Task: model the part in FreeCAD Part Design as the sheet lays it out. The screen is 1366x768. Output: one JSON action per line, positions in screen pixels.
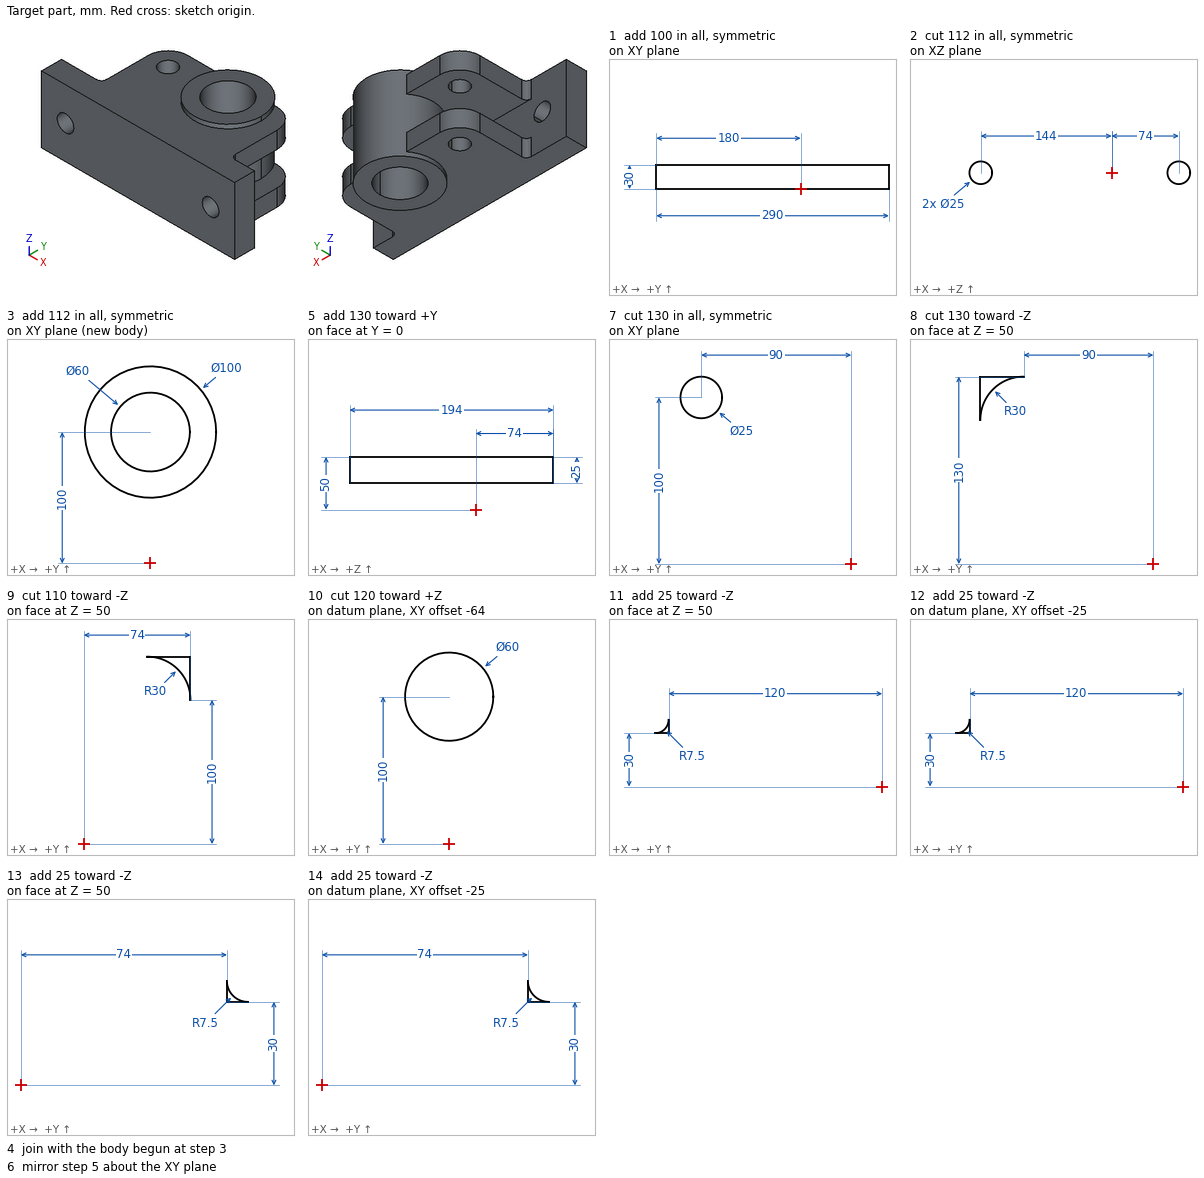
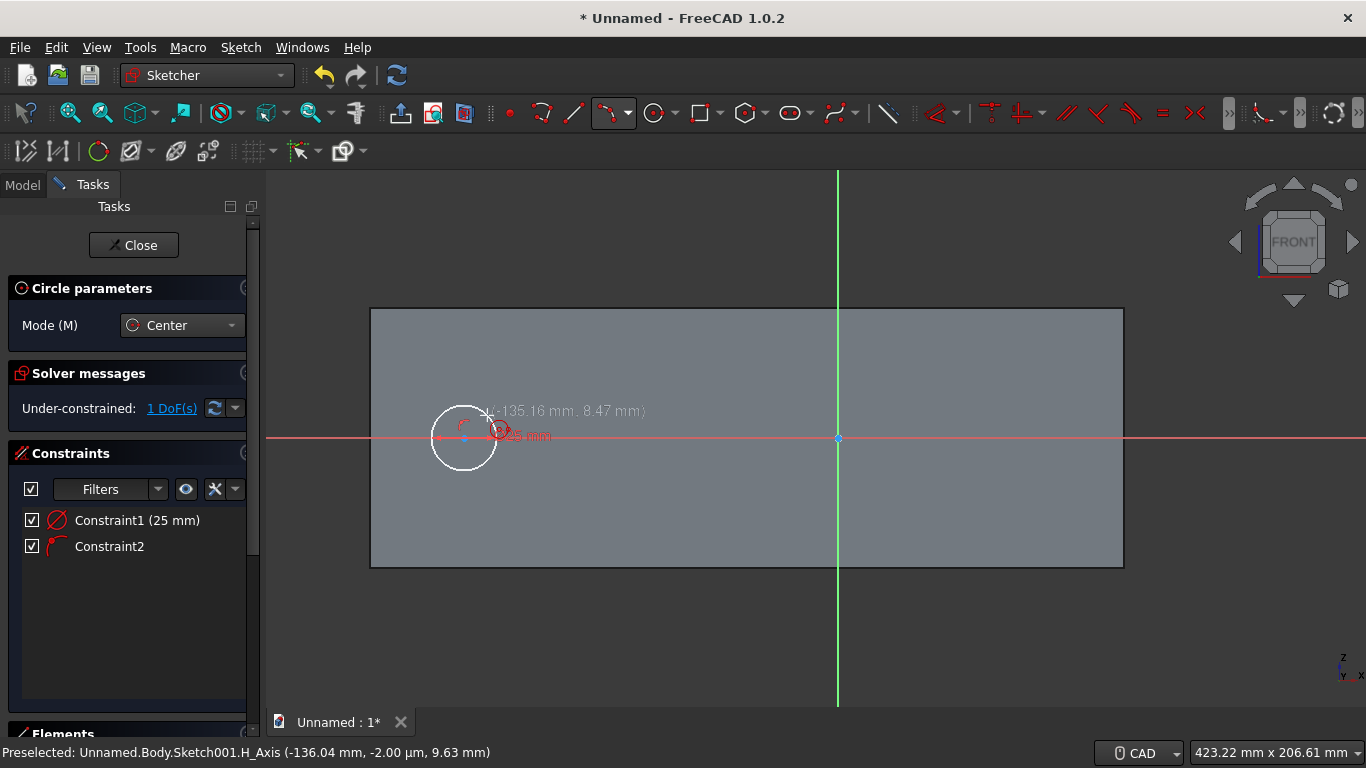
{"action": "left_click", "coordinate": [1031, 438]}
{"action": "mouse_move", "coordinate": [1054, 415]}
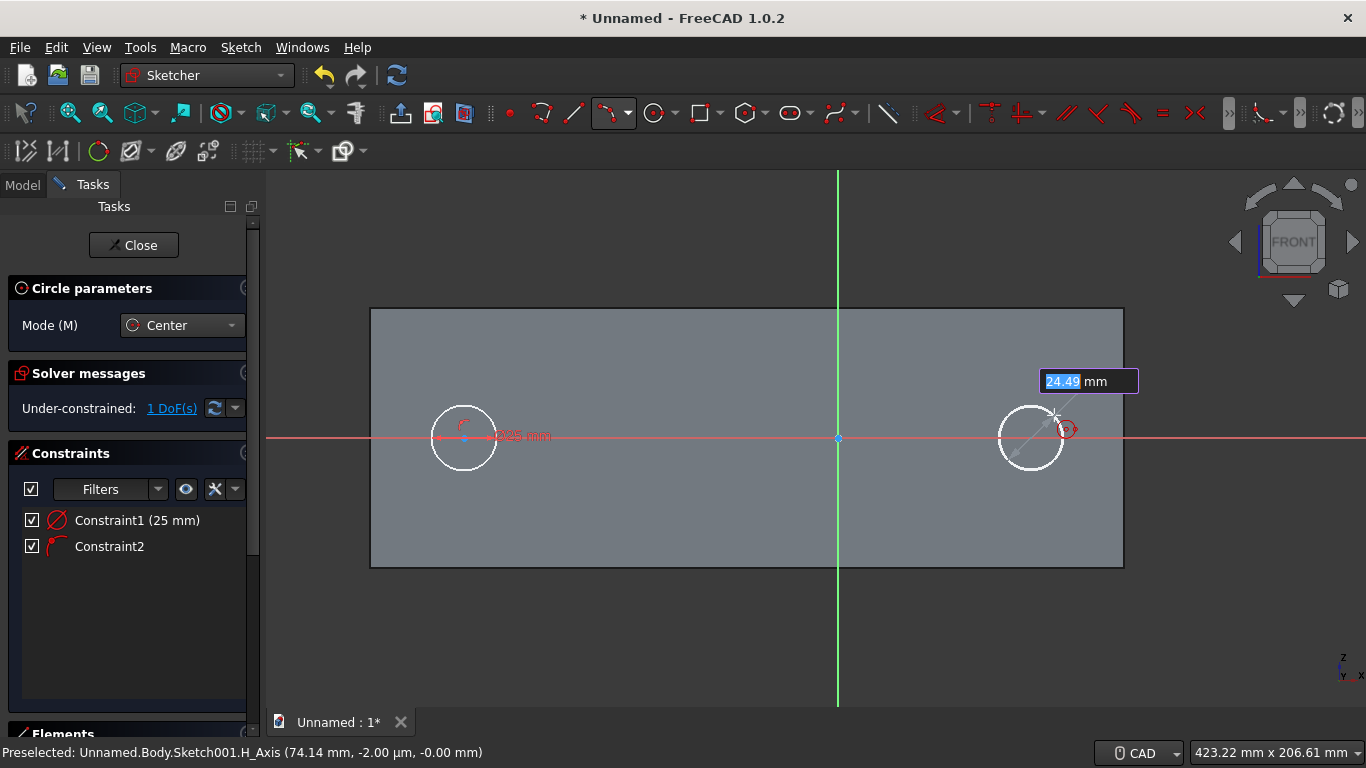
{"action": "type", "text": "25"}
{"action": "key", "text": "Return"}
{"action": "key", "text": "Escape"}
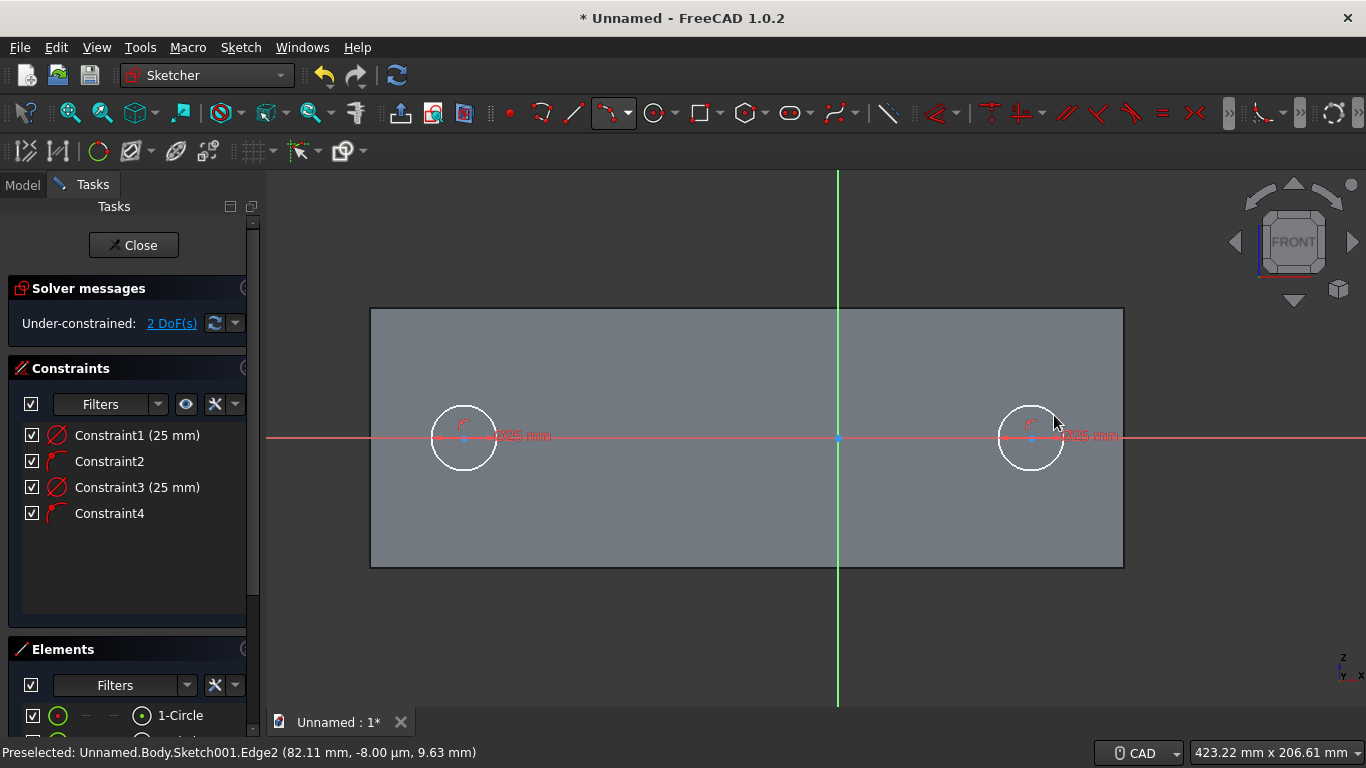
{"action": "left_click", "coordinate": [936, 114]}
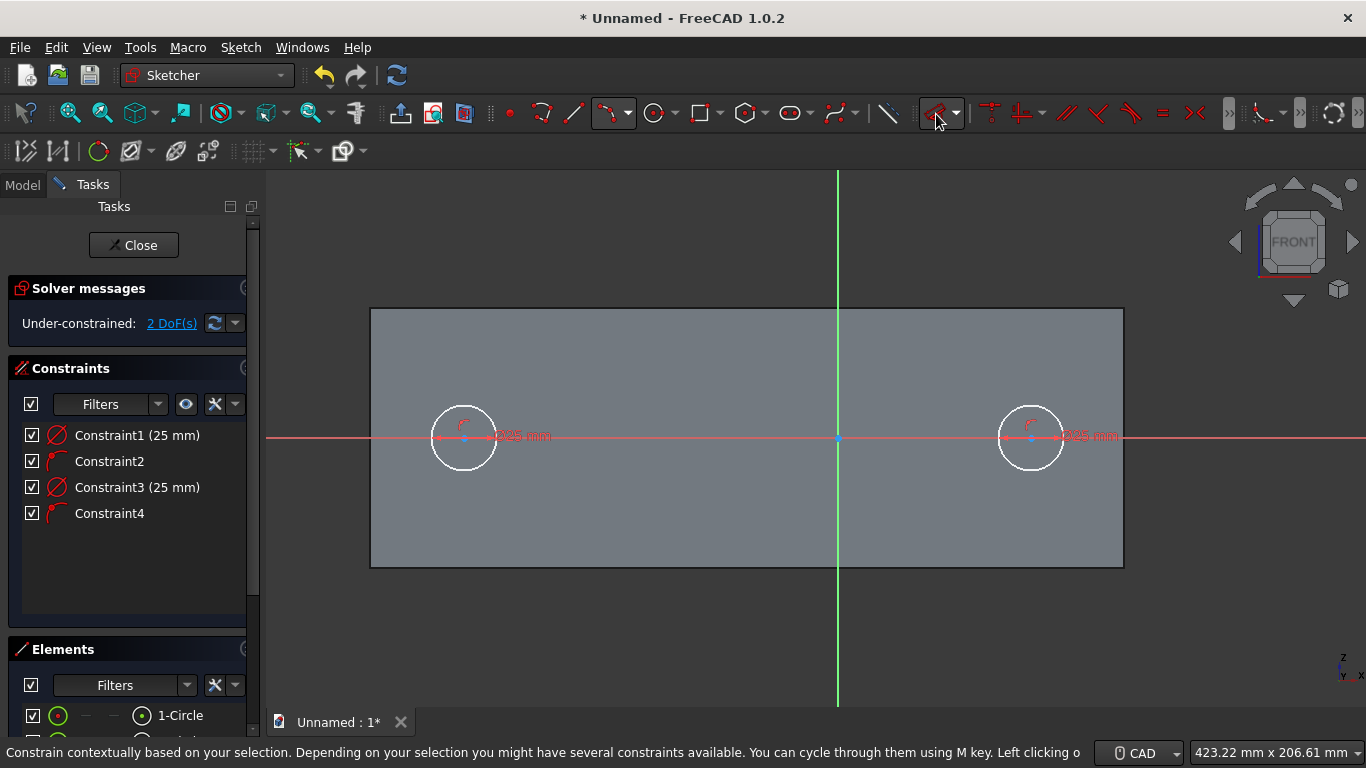
{"action": "left_click", "coordinate": [1031, 438]}
{"action": "left_click", "coordinate": [935, 472]}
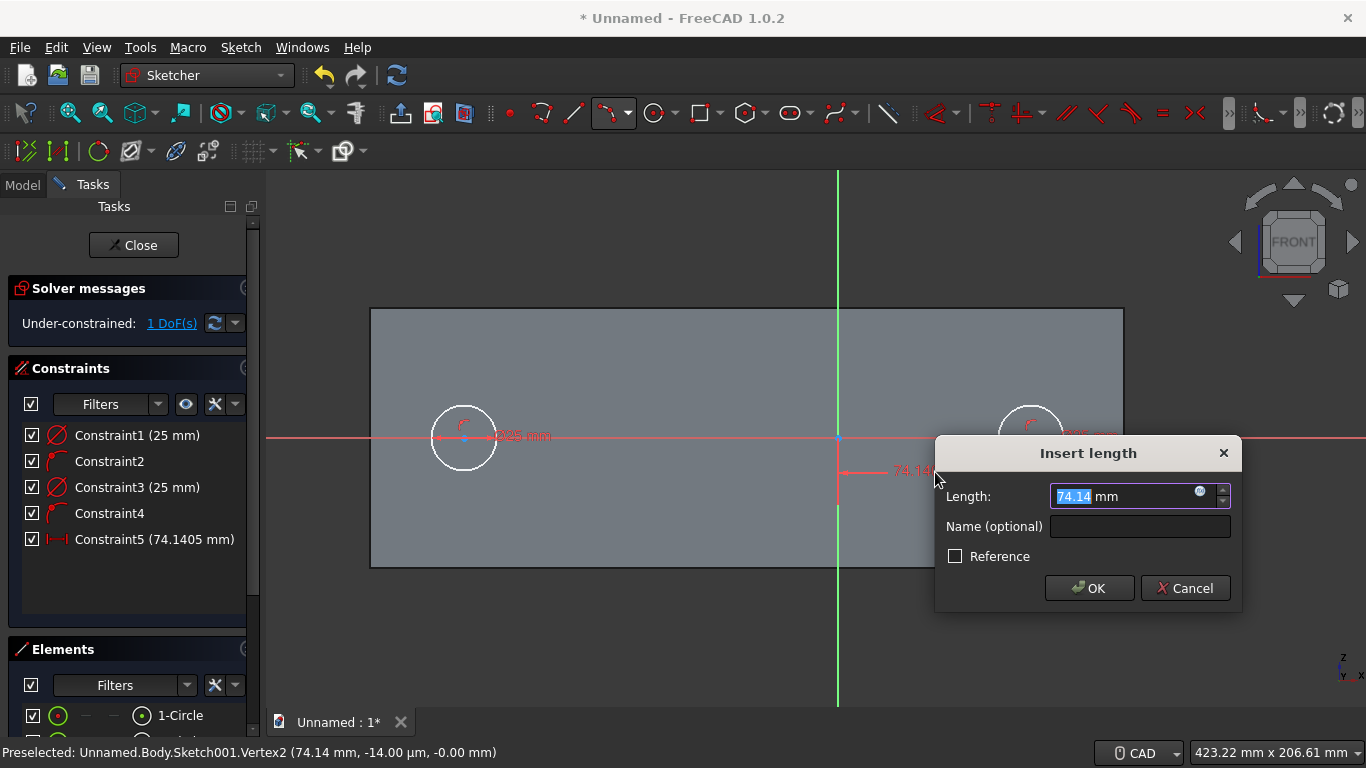
{"action": "type", "text": "74"}
{"action": "key", "text": "Return"}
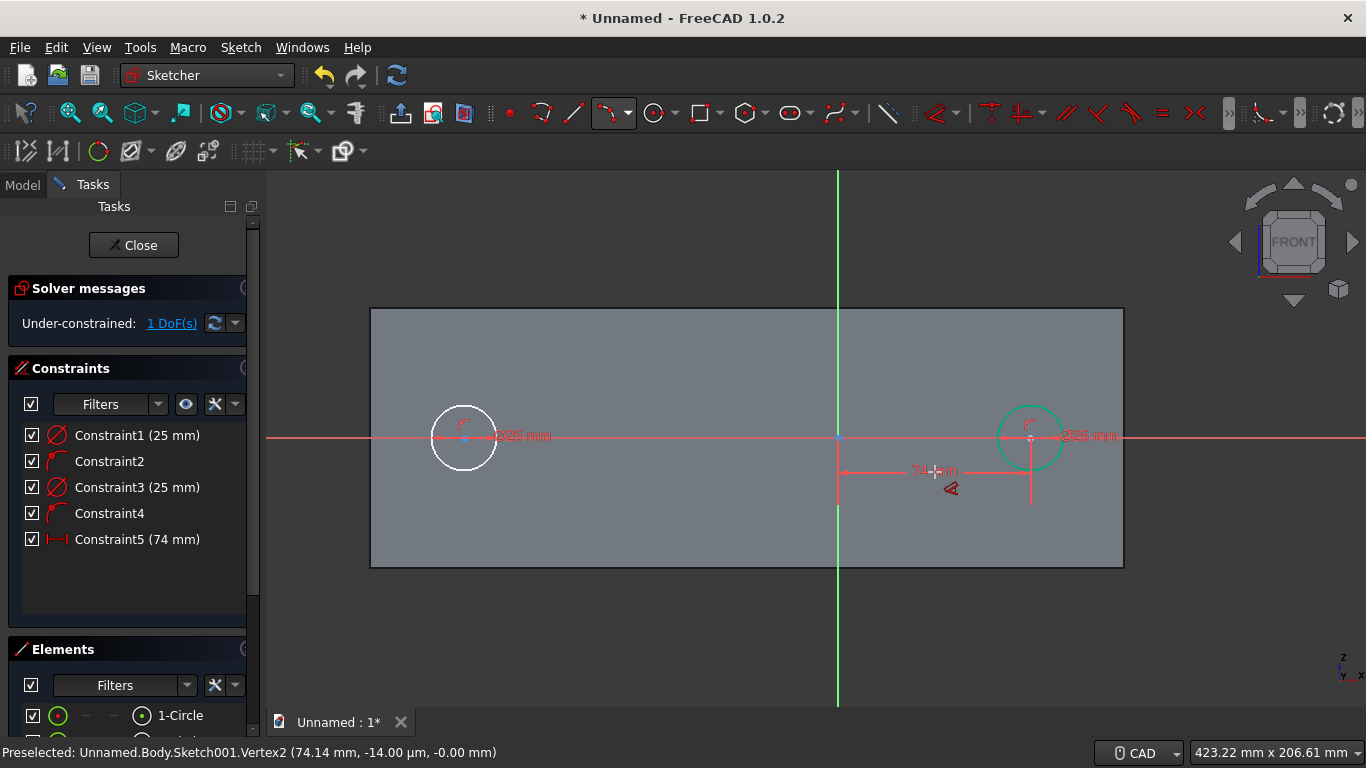
{"action": "left_click", "coordinate": [464, 438]}
{"action": "left_click", "coordinate": [651, 472]}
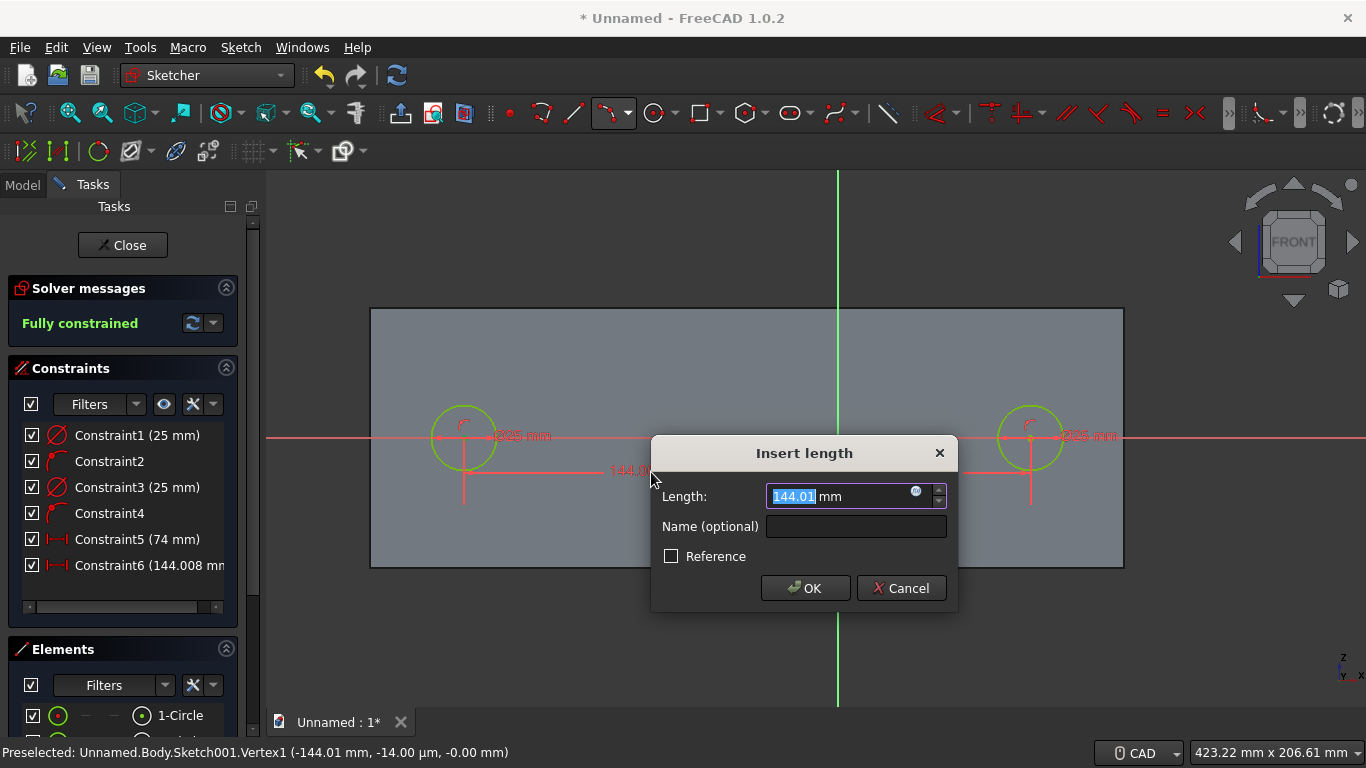
{"action": "type", "text": "144"}
{"action": "key", "text": "Return"}
{"action": "key", "text": "Escape"}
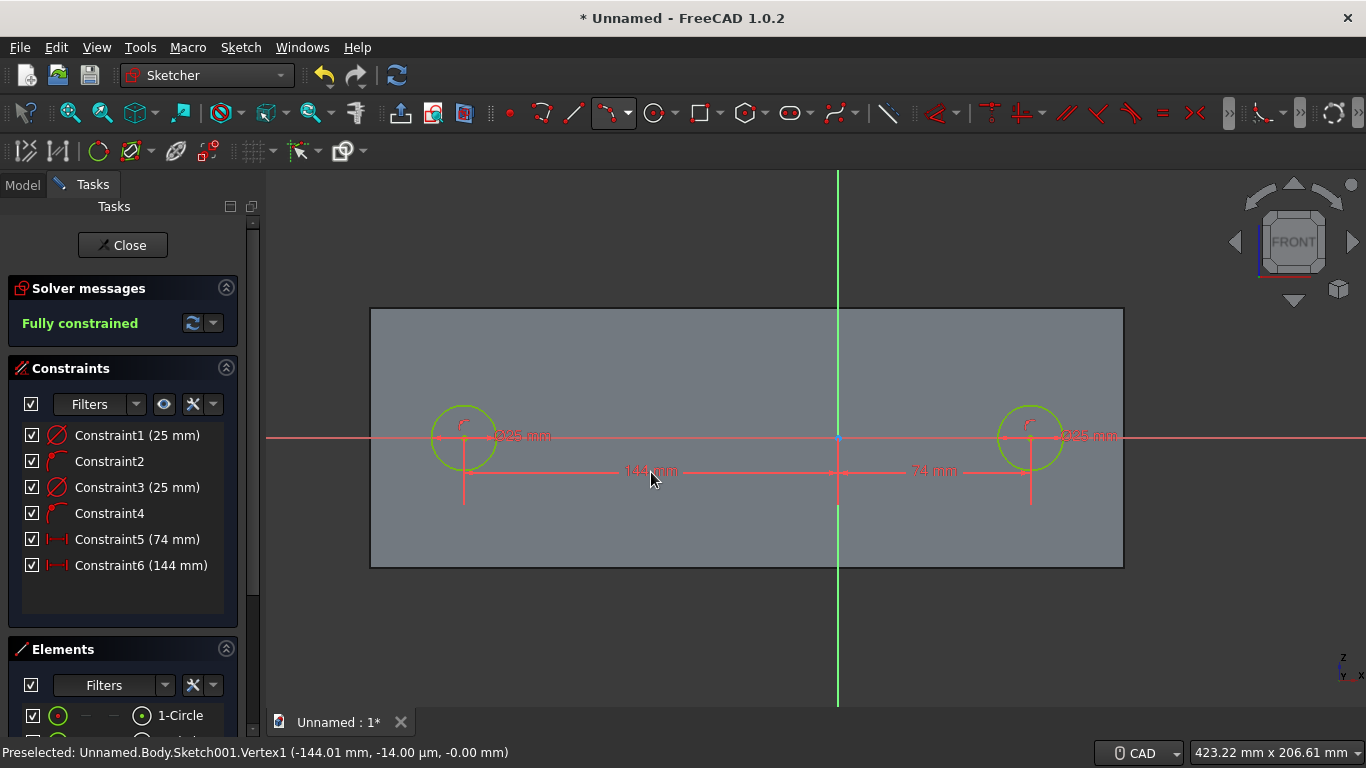
{"action": "left_click", "coordinate": [123, 245]}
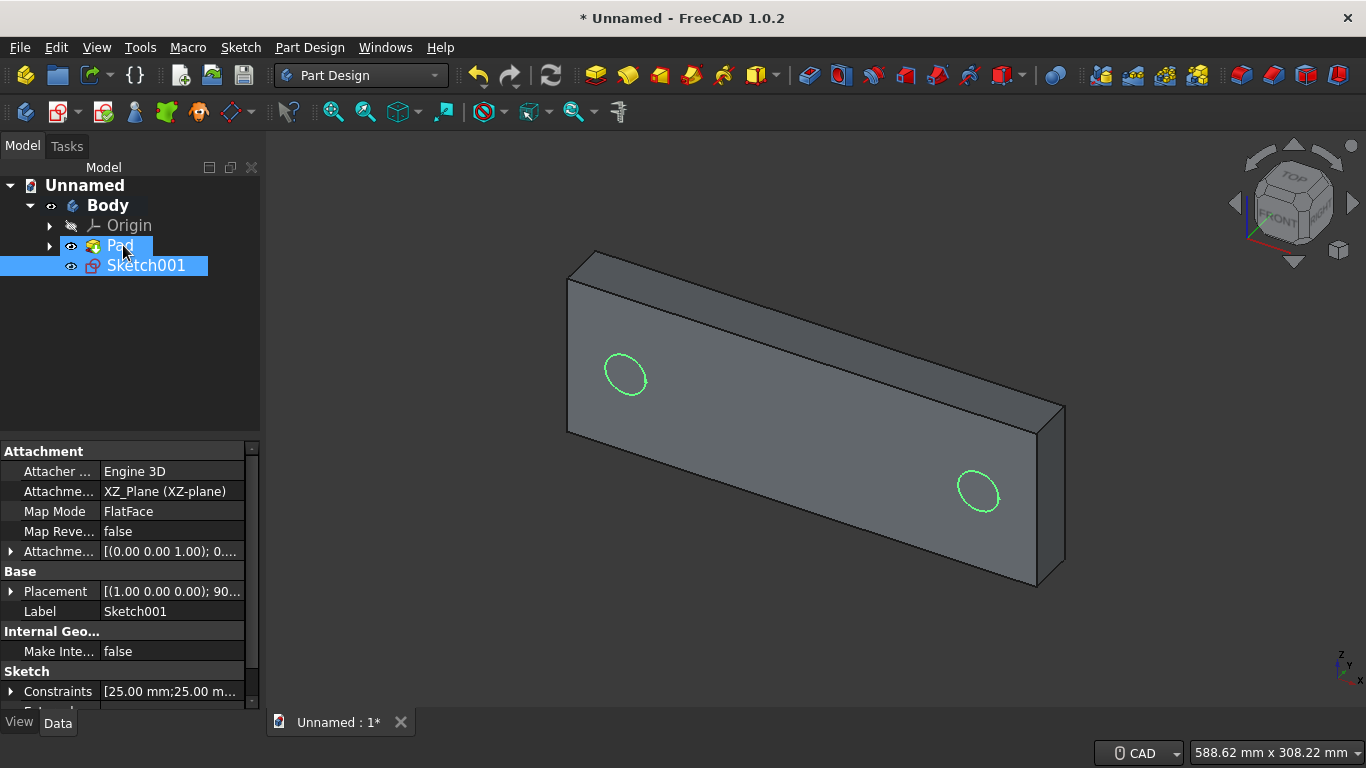
{"action": "left_click", "coordinate": [810, 76]}